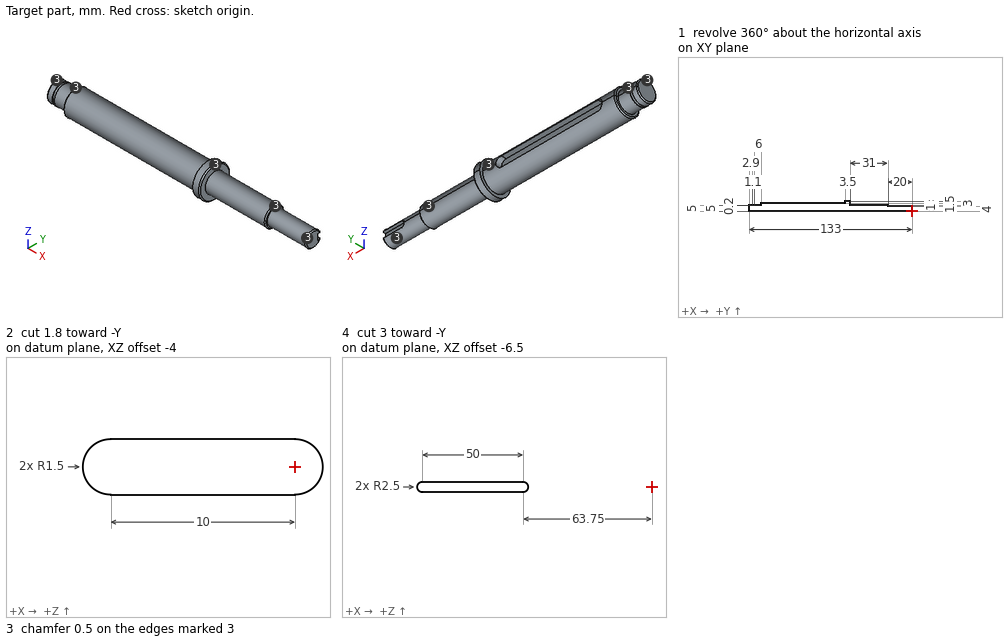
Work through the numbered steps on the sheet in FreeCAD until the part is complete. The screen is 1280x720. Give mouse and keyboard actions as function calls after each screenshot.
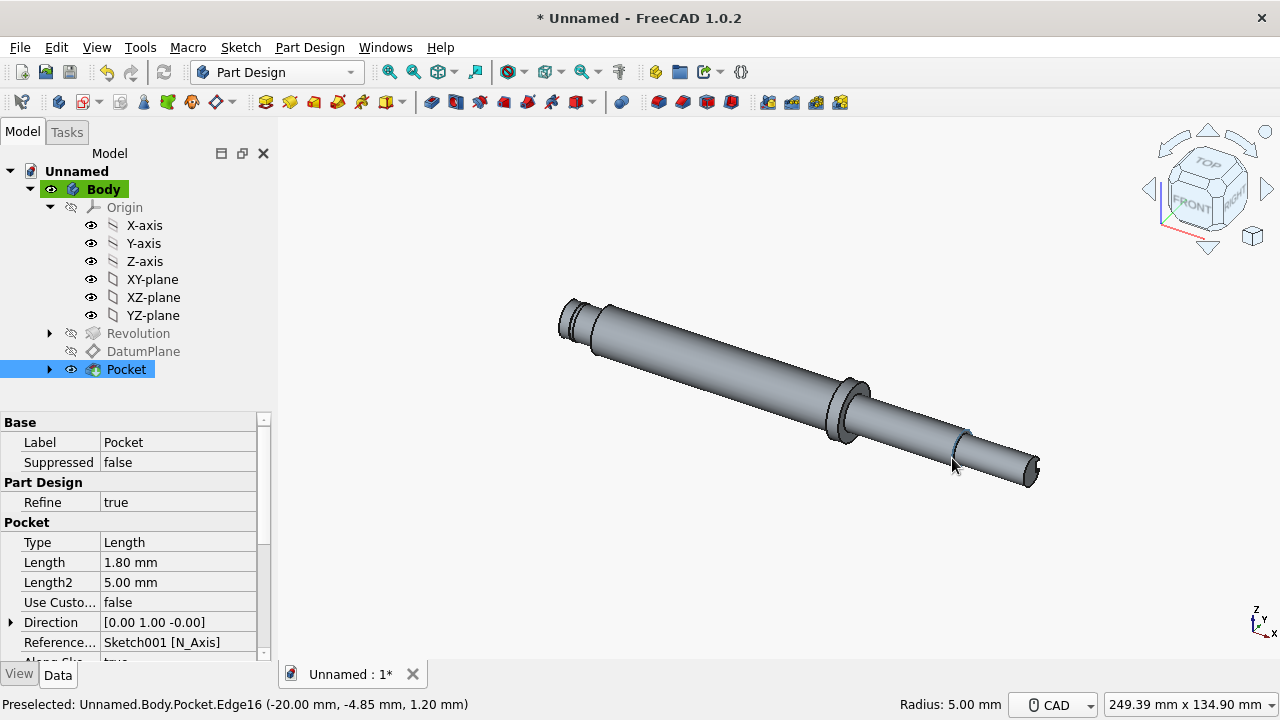
click(838, 428, ctrl)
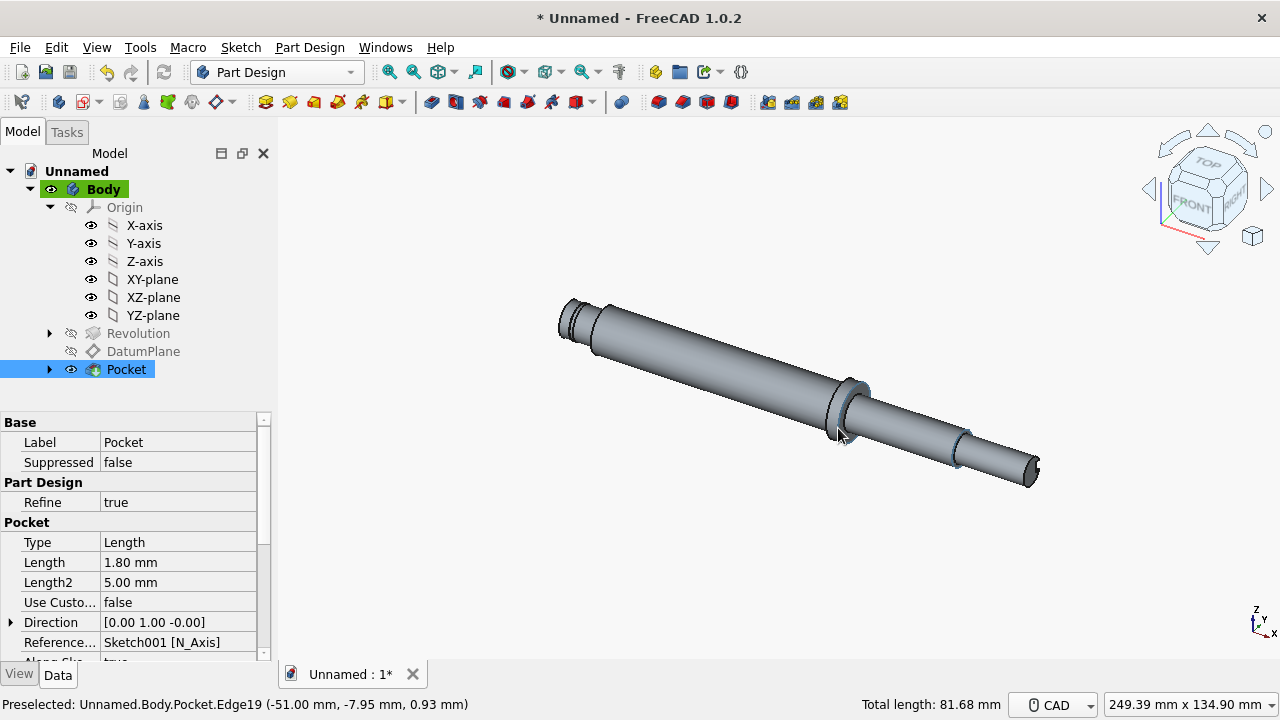
click(608, 305, ctrl)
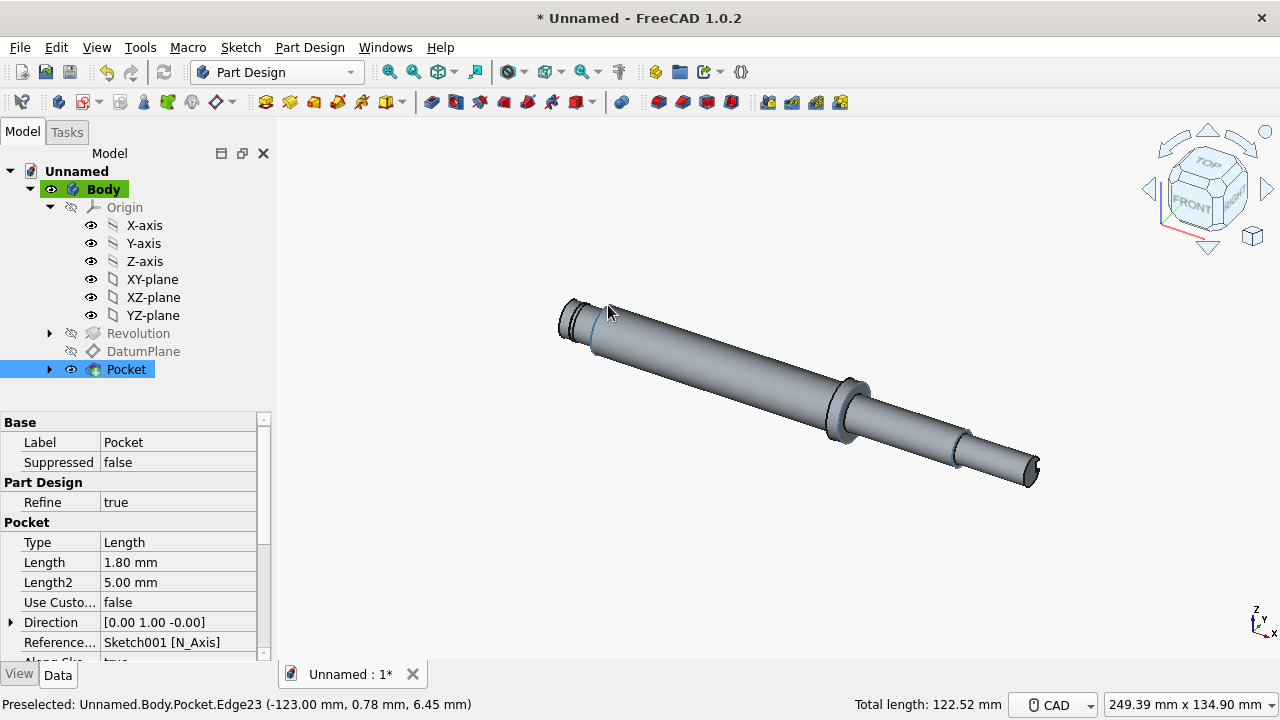
click(559, 327, ctrl)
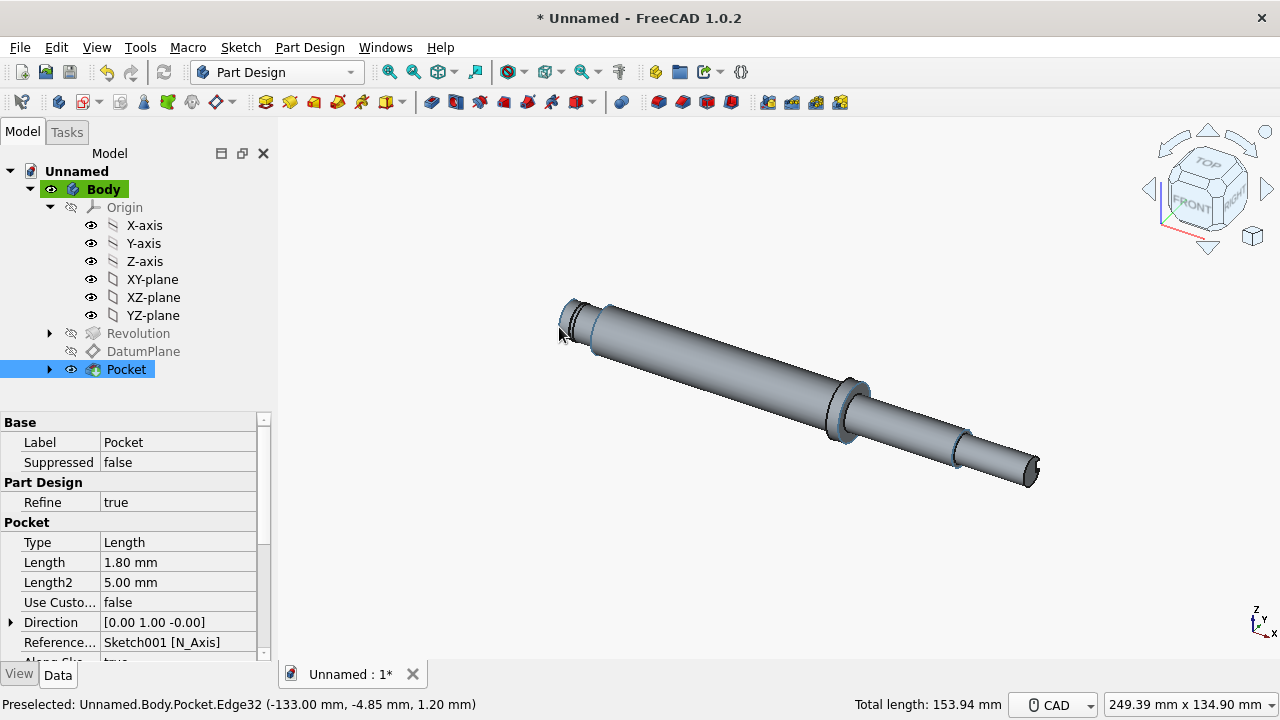
click(1024, 479, ctrl)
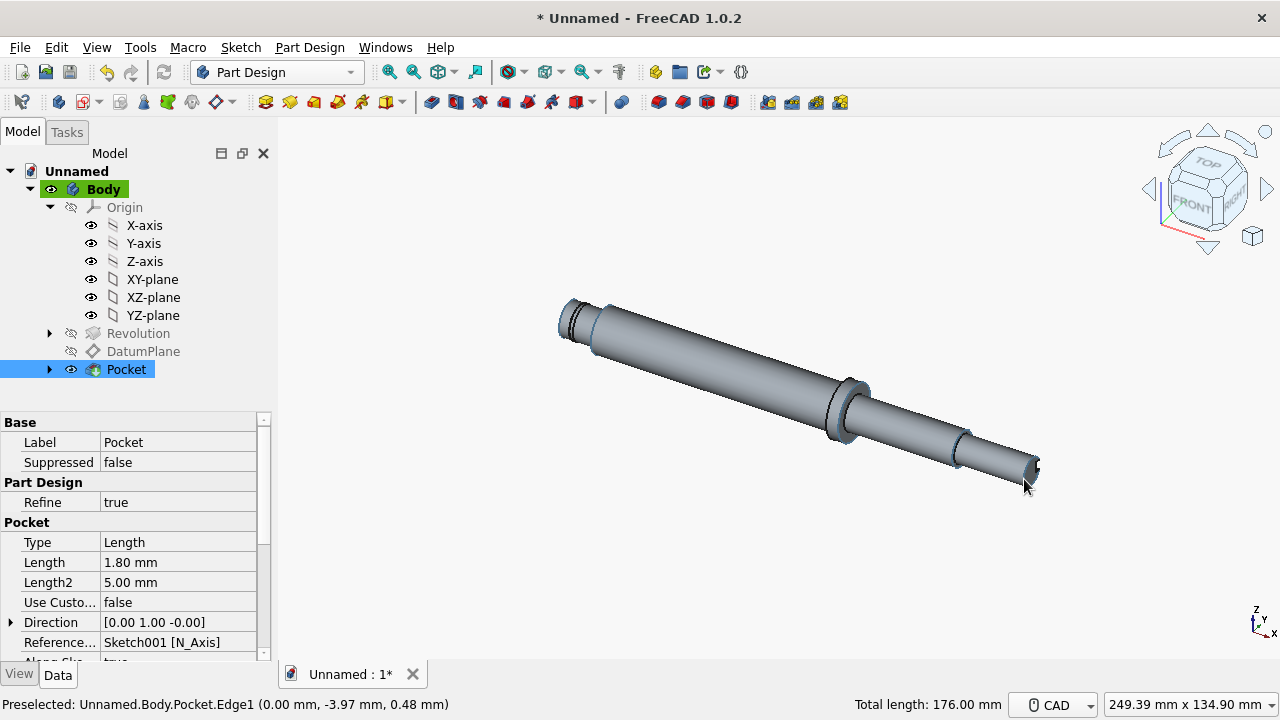
click(684, 102)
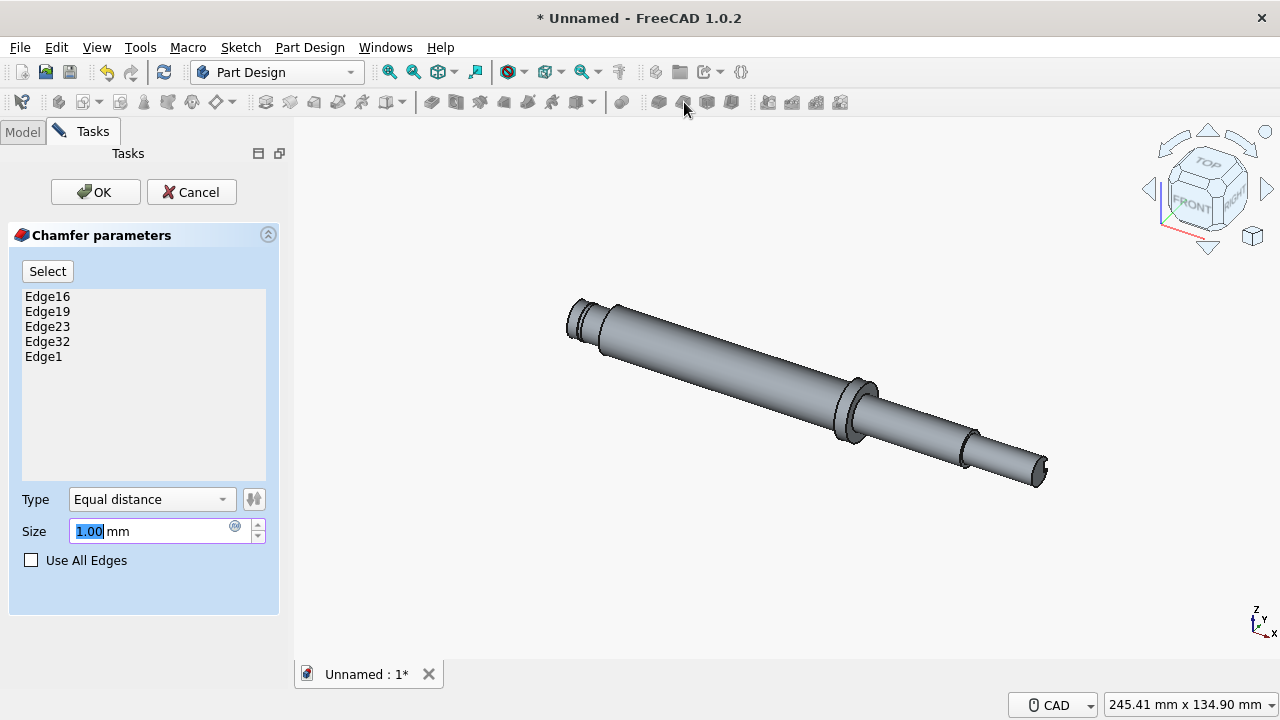
text(0.5)
key(Tab)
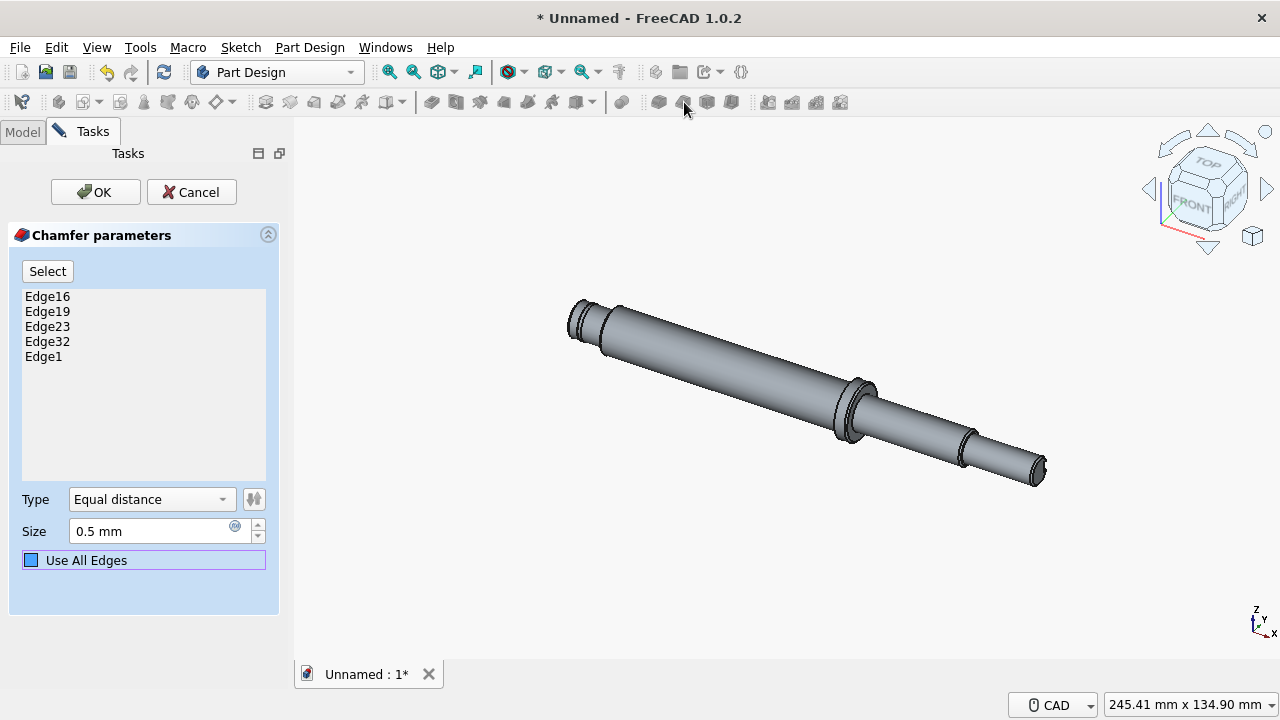
click(96, 192)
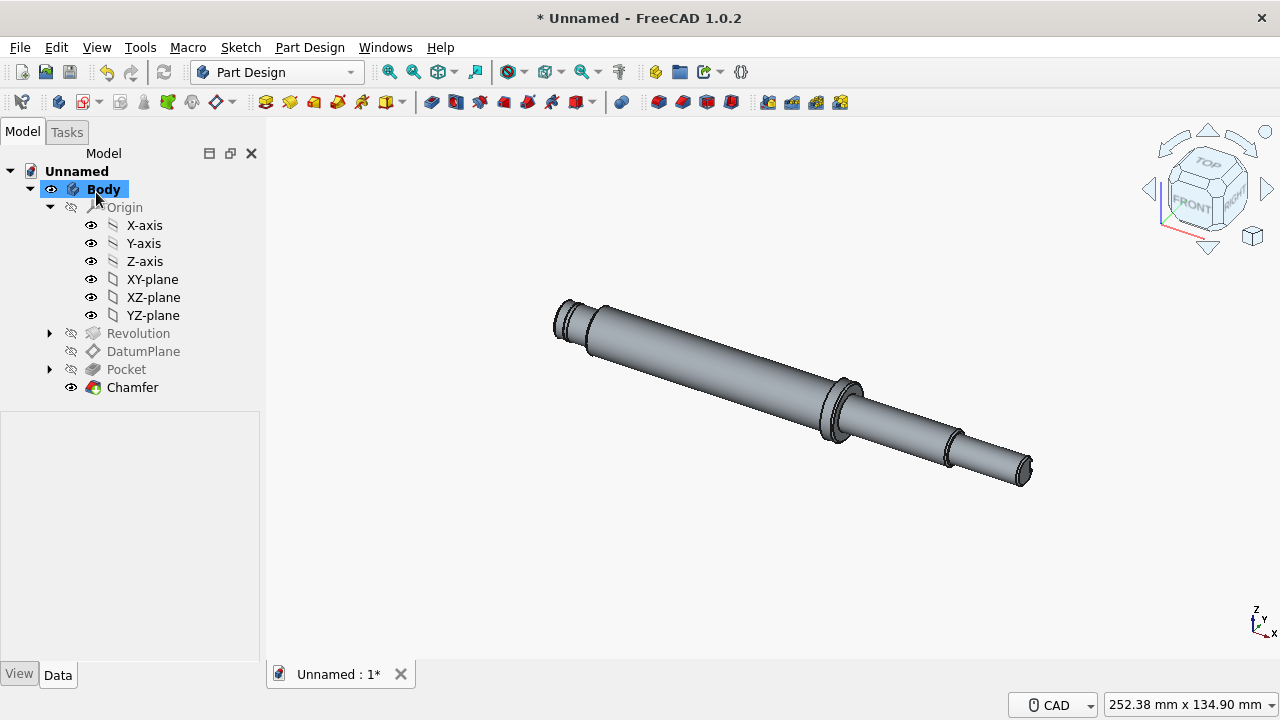
click(136, 297)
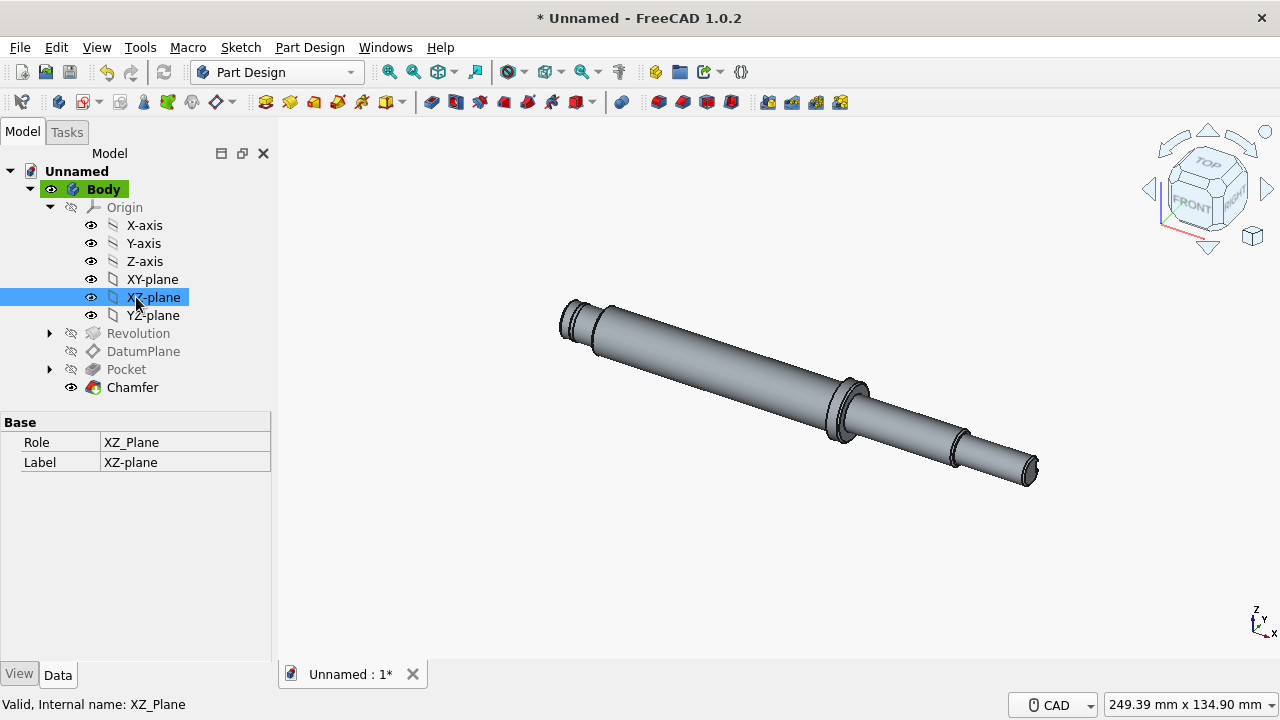
click(216, 102)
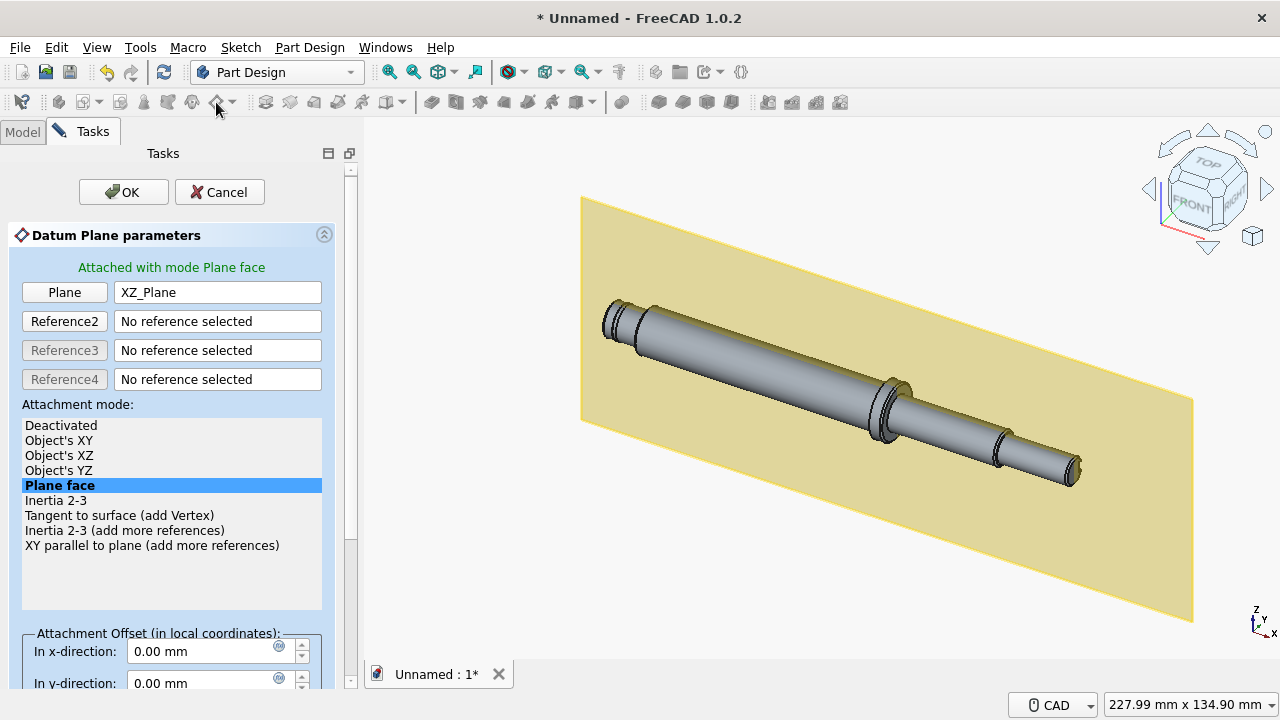
scroll(351, 426, down, 2)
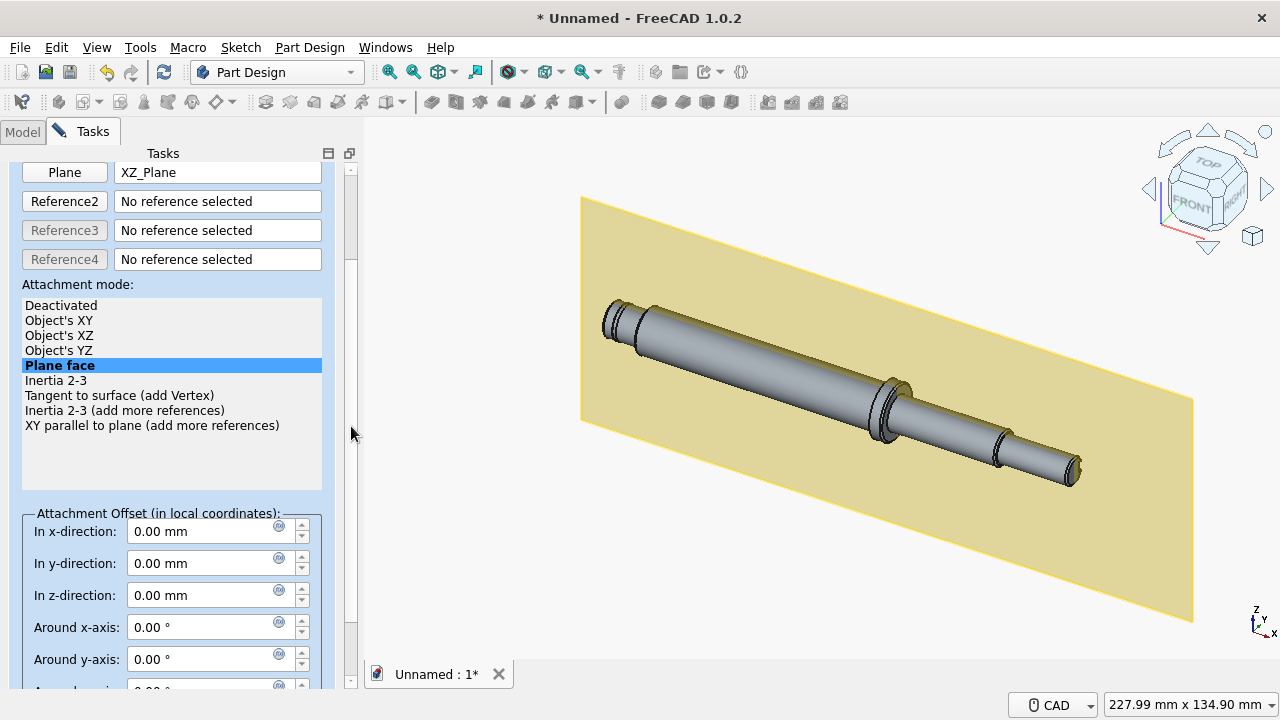
triple_click(210, 595)